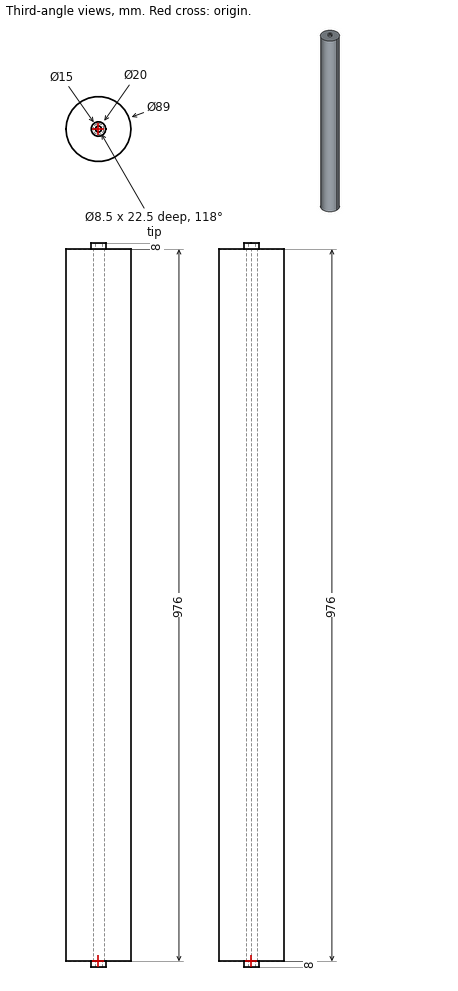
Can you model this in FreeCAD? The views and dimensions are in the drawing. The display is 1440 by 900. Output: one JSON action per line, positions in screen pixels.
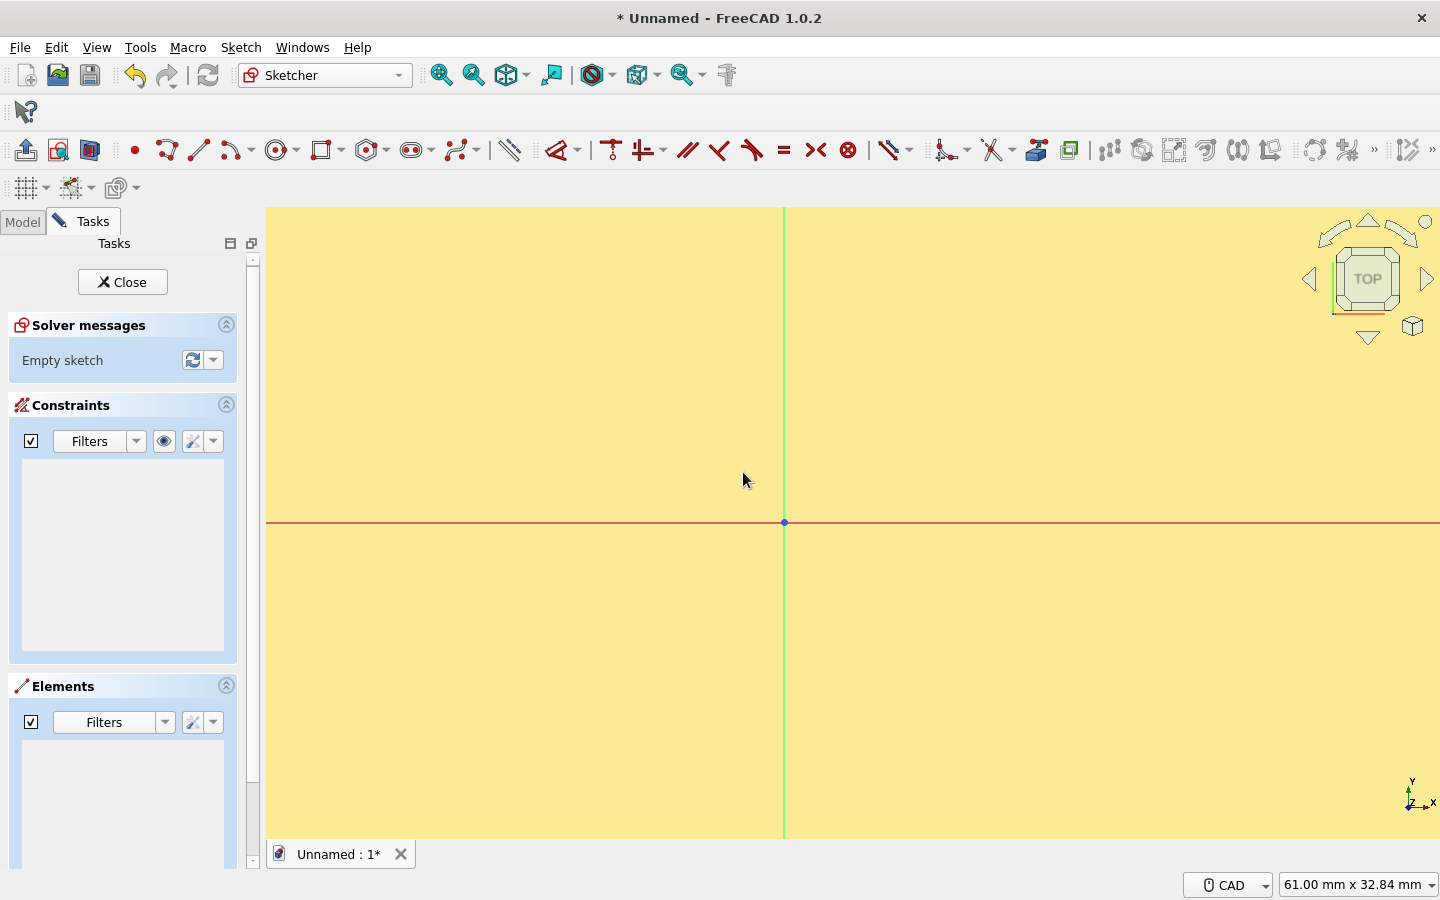
{"action": "left_click", "coordinate": [276, 150]}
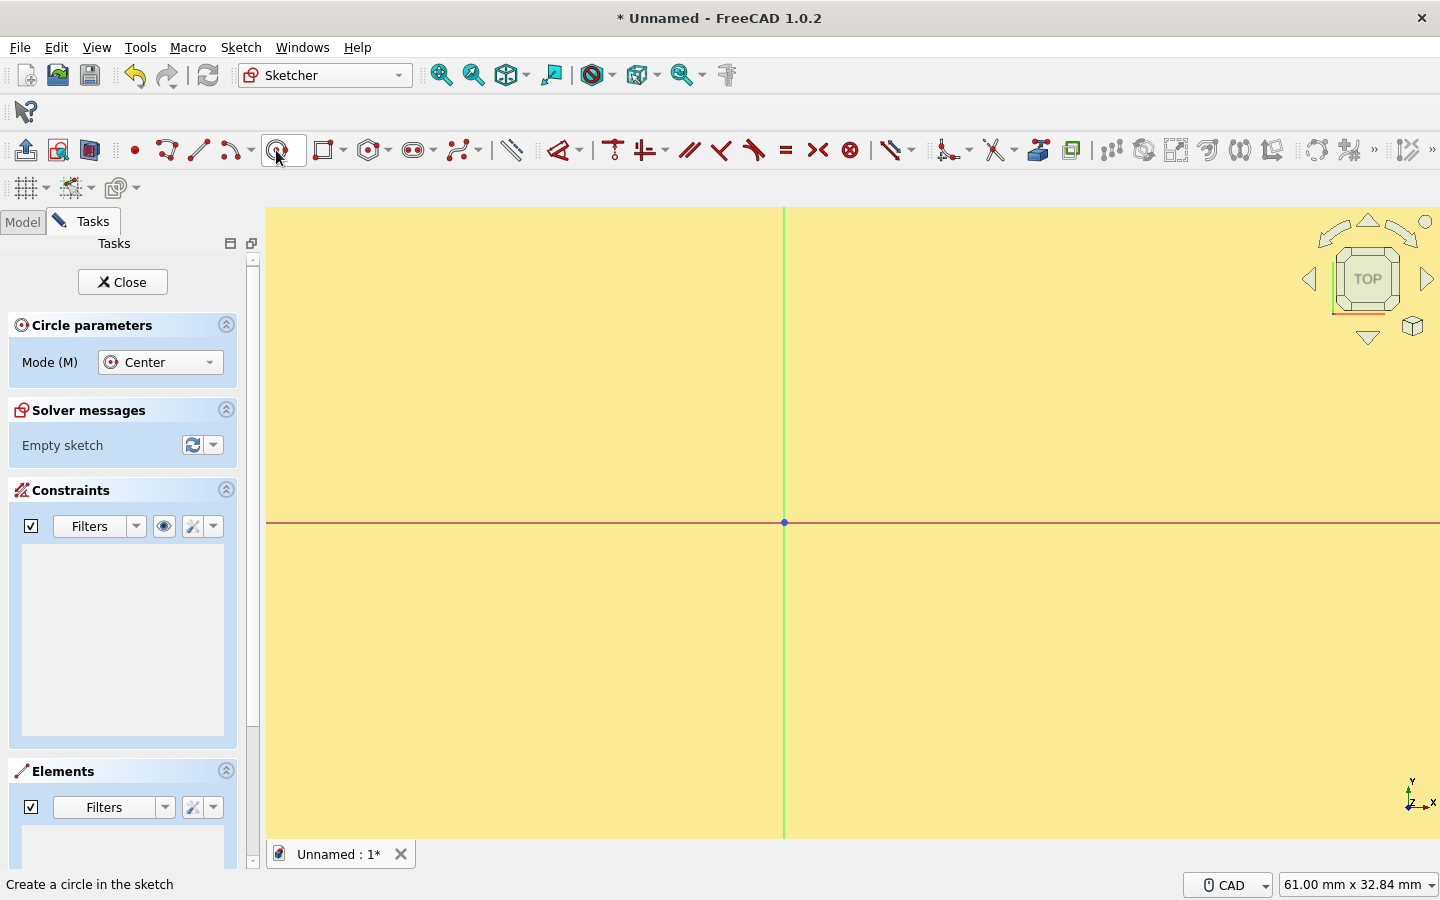
{"action": "left_click", "coordinate": [784, 523]}
{"action": "left_click", "coordinate": [920, 387]}
{"action": "key", "text": "Escape"}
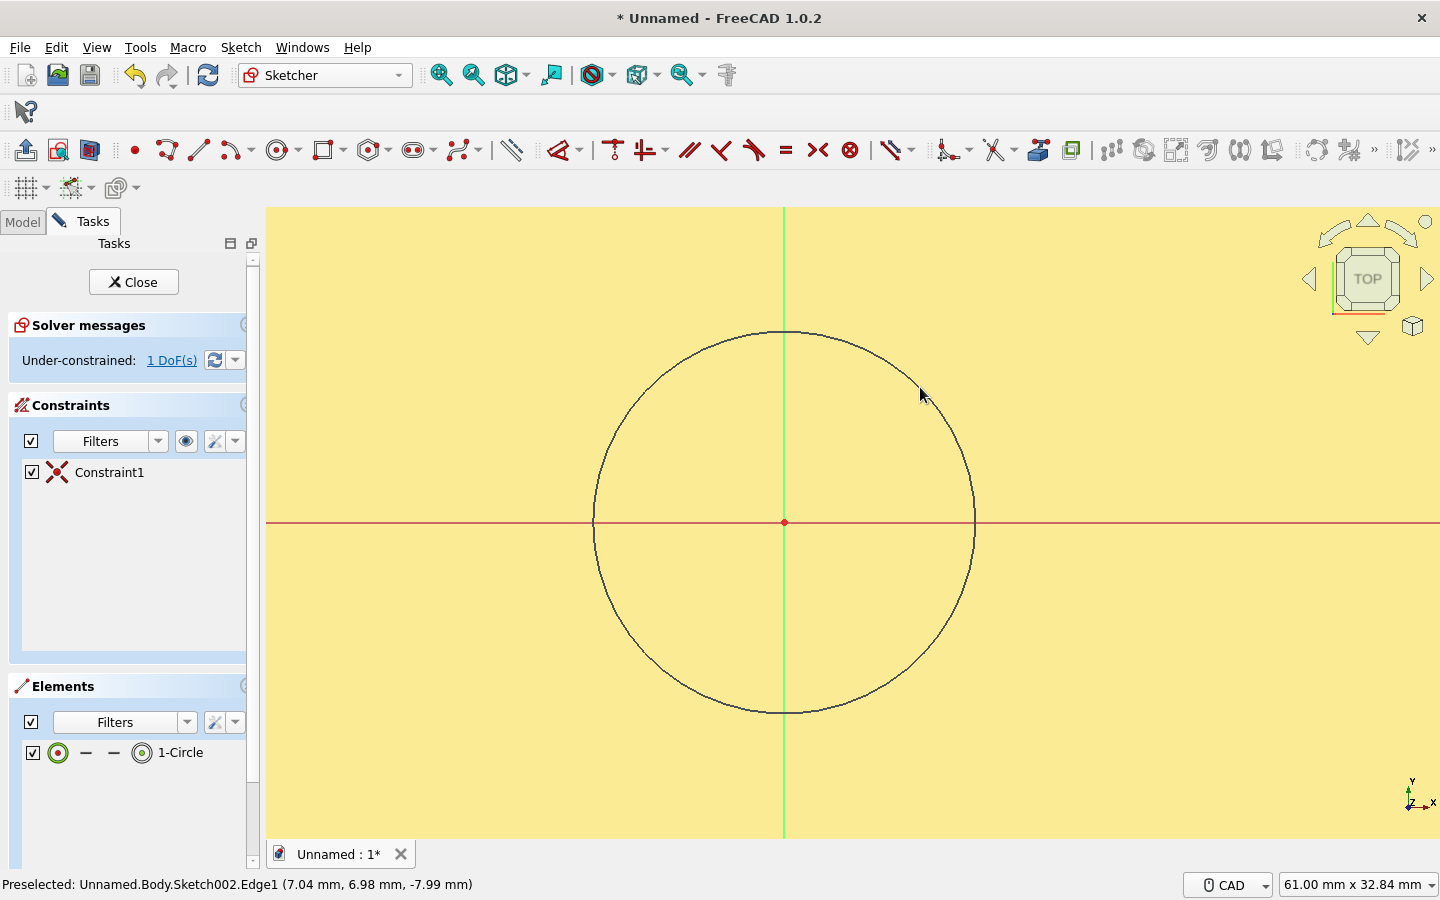
{"action": "left_click", "coordinate": [558, 150]}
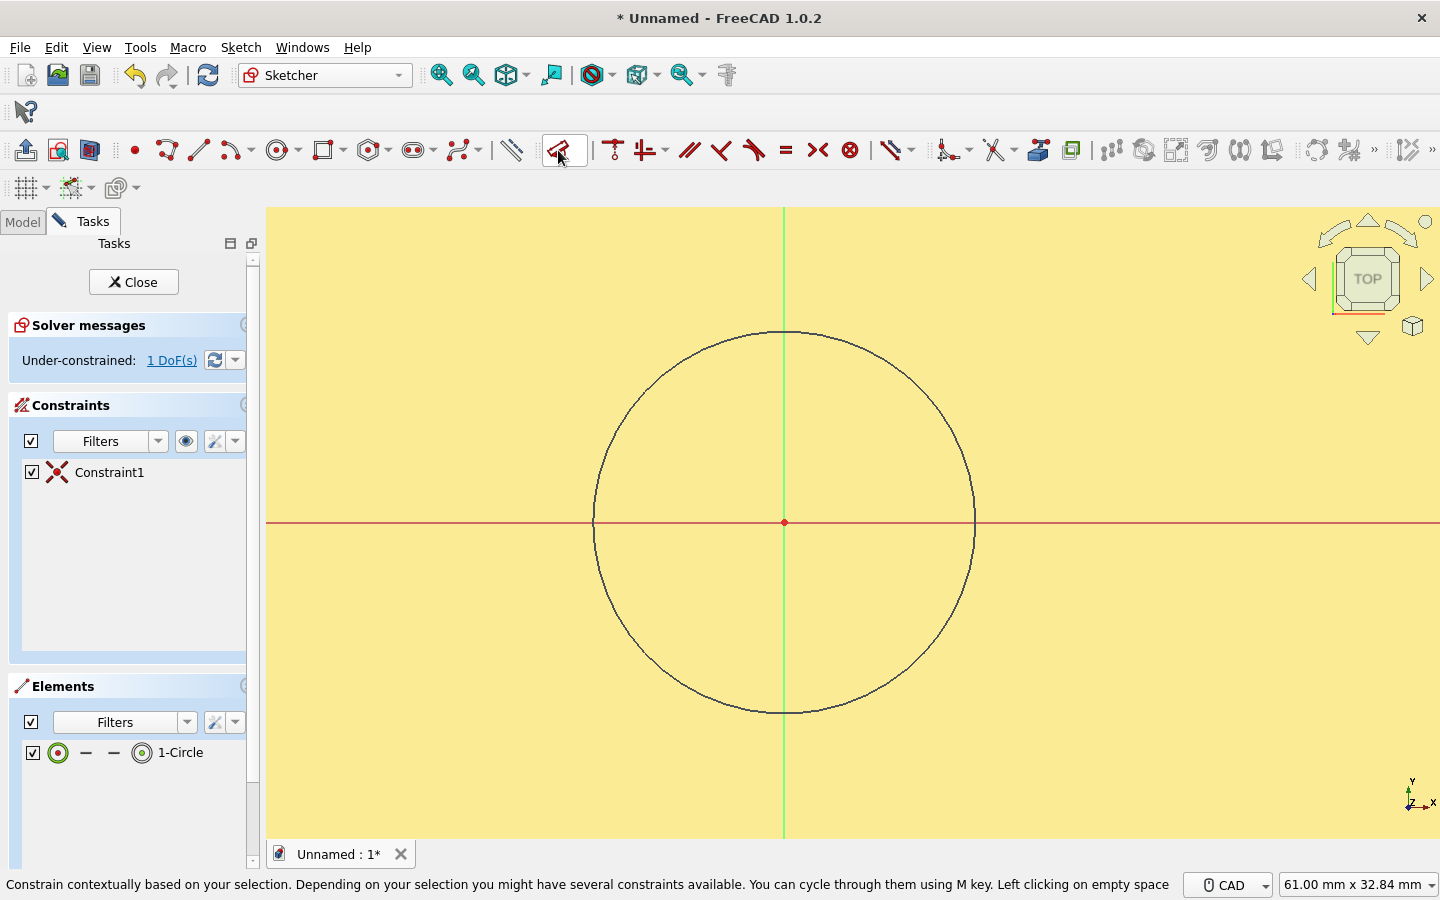
{"action": "left_click", "coordinate": [919, 387]}
{"action": "left_click", "coordinate": [942, 364]}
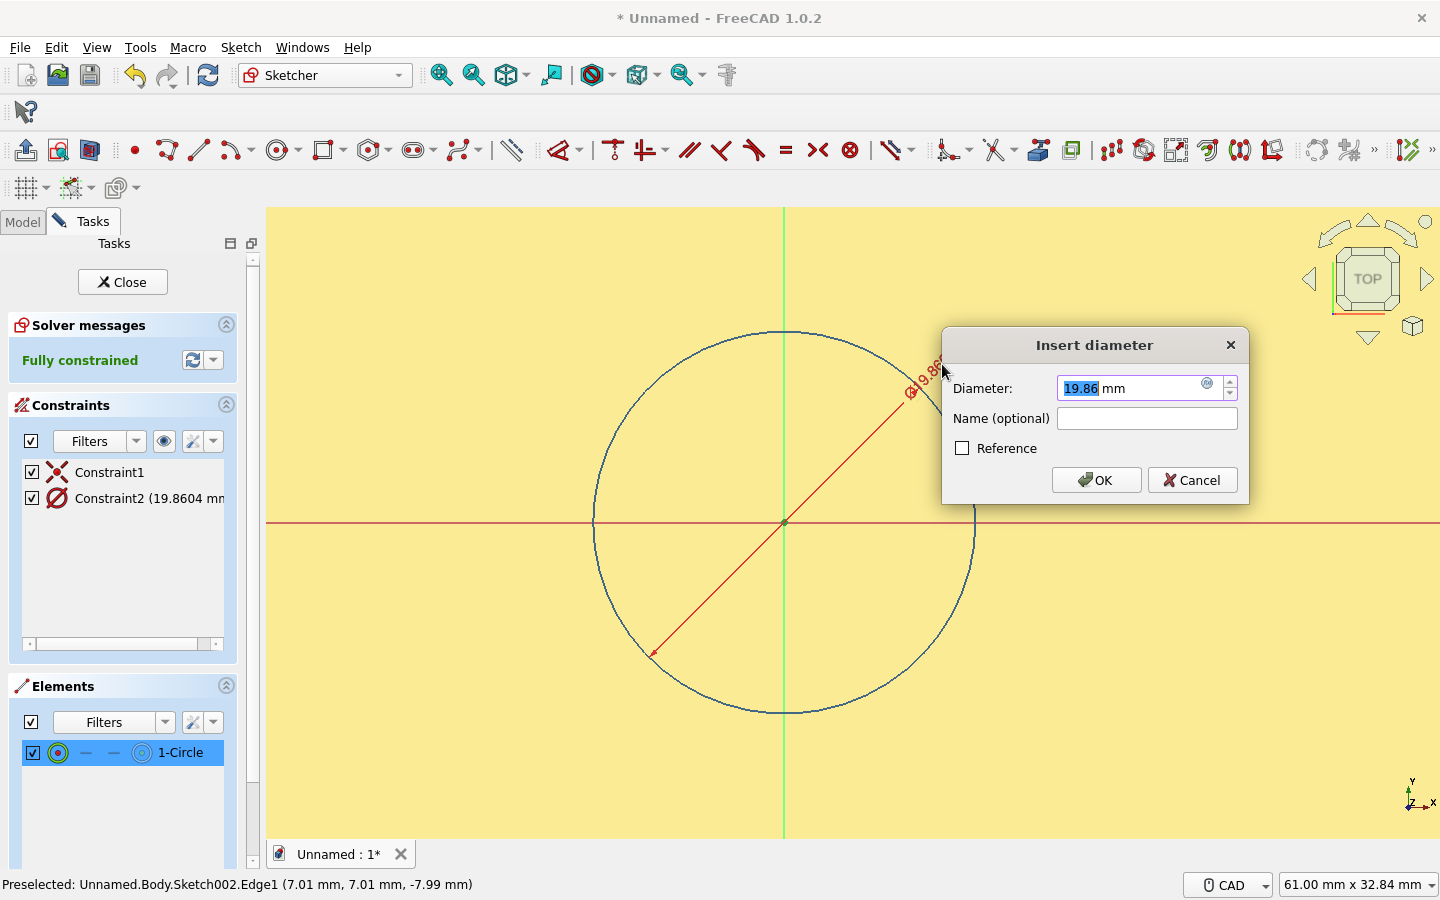
{"action": "type", "text": "20"}
{"action": "key", "text": "Return"}
{"action": "key", "text": "Escape"}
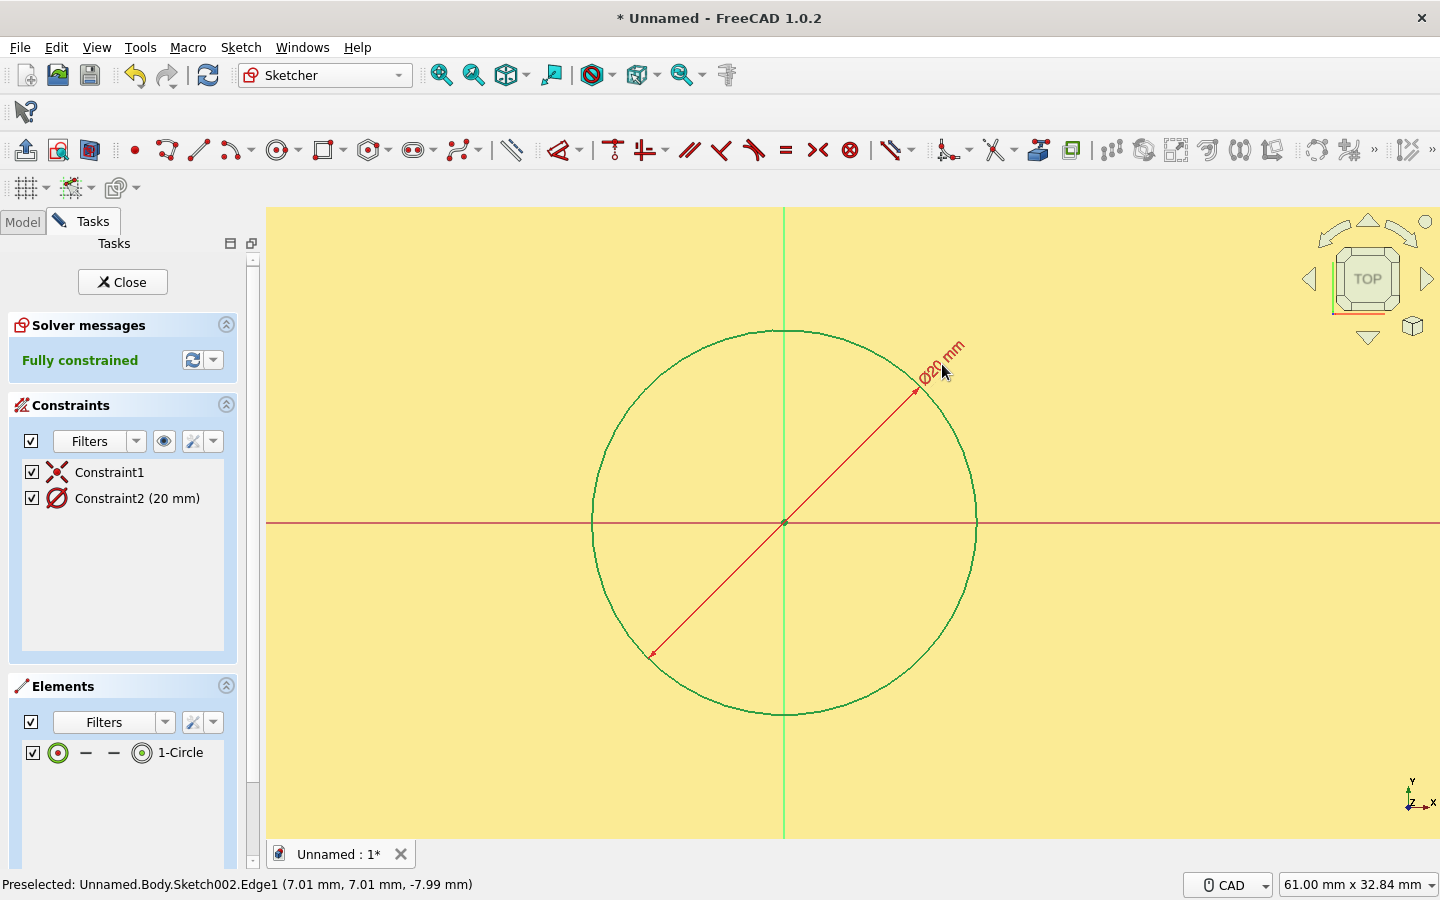
{"action": "left_click", "coordinate": [123, 282]}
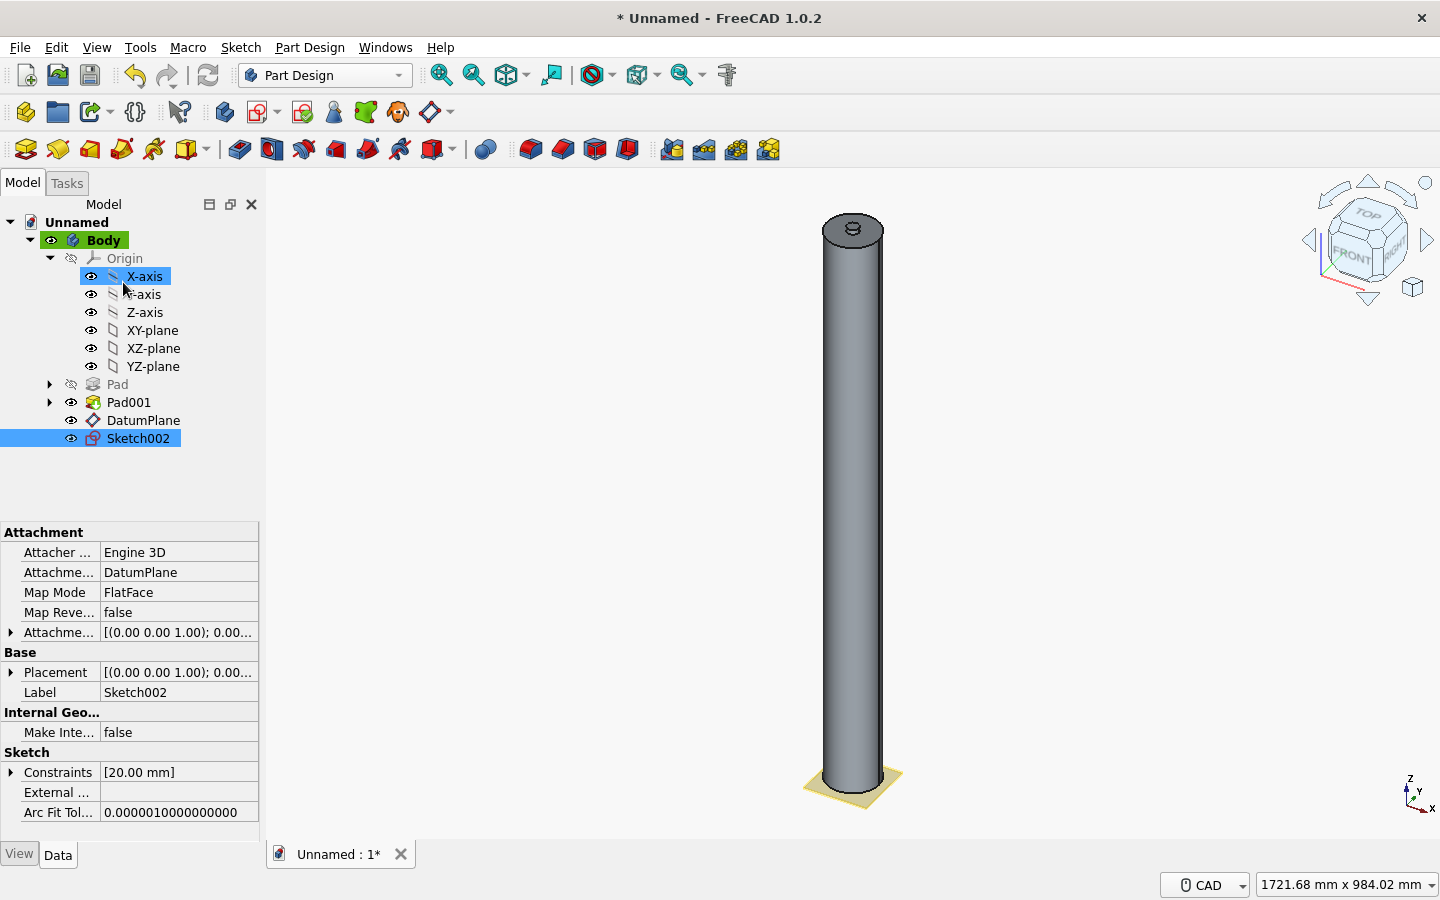
{"action": "left_click", "coordinate": [26, 150]}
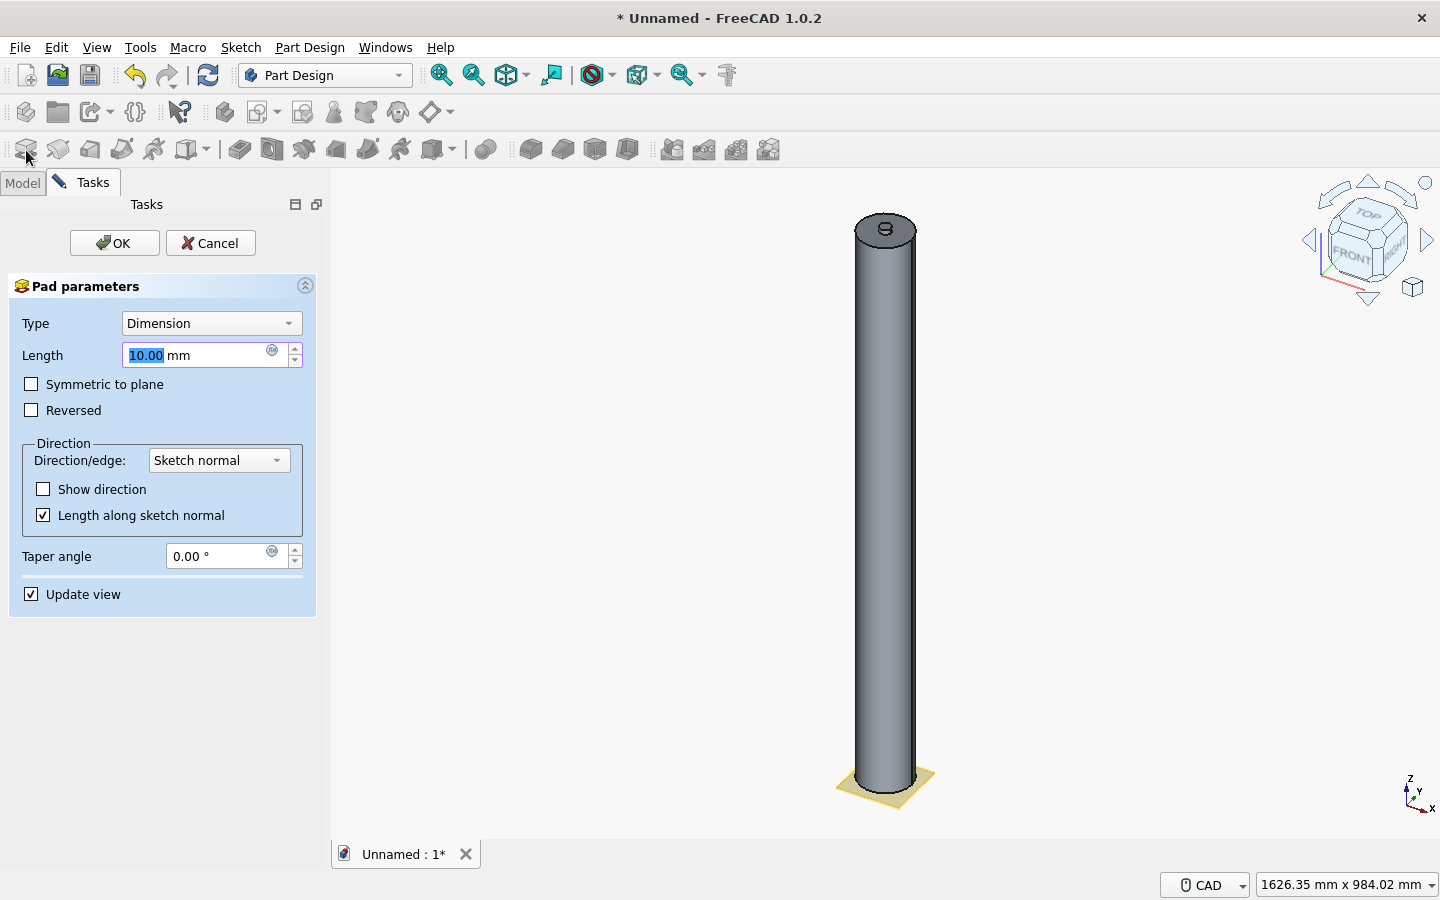
{"action": "type", "text": "8"}
{"action": "key", "text": "Tab"}